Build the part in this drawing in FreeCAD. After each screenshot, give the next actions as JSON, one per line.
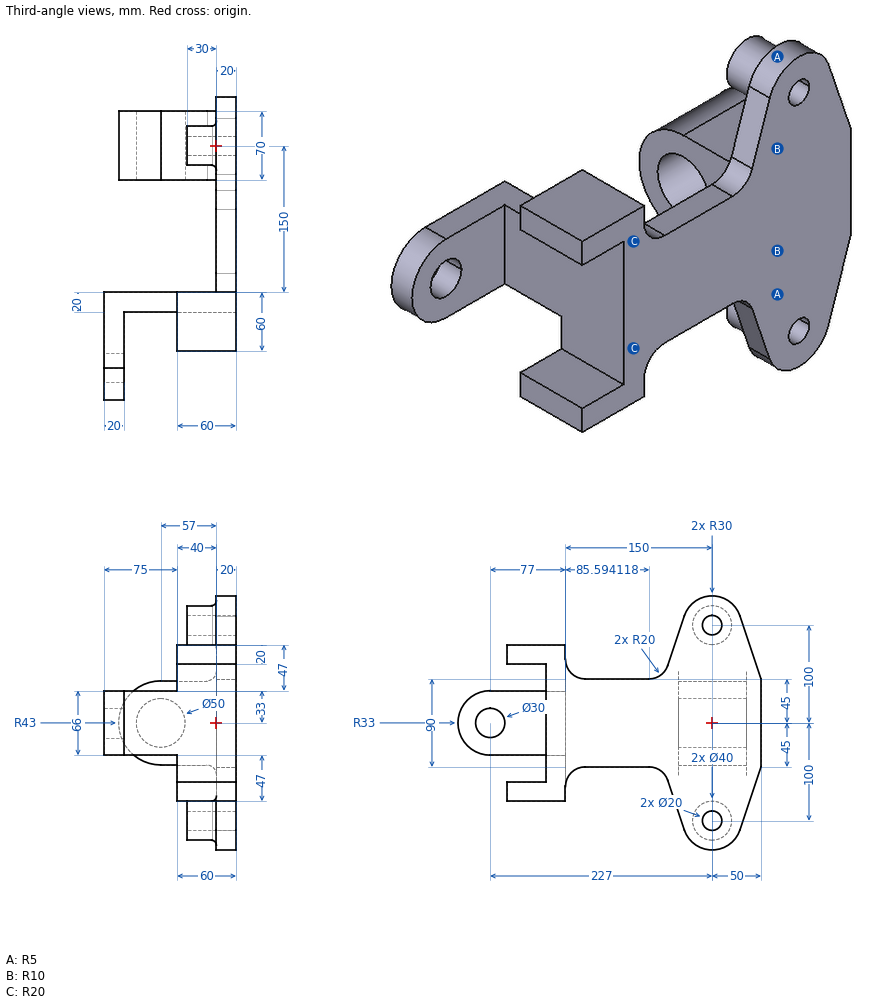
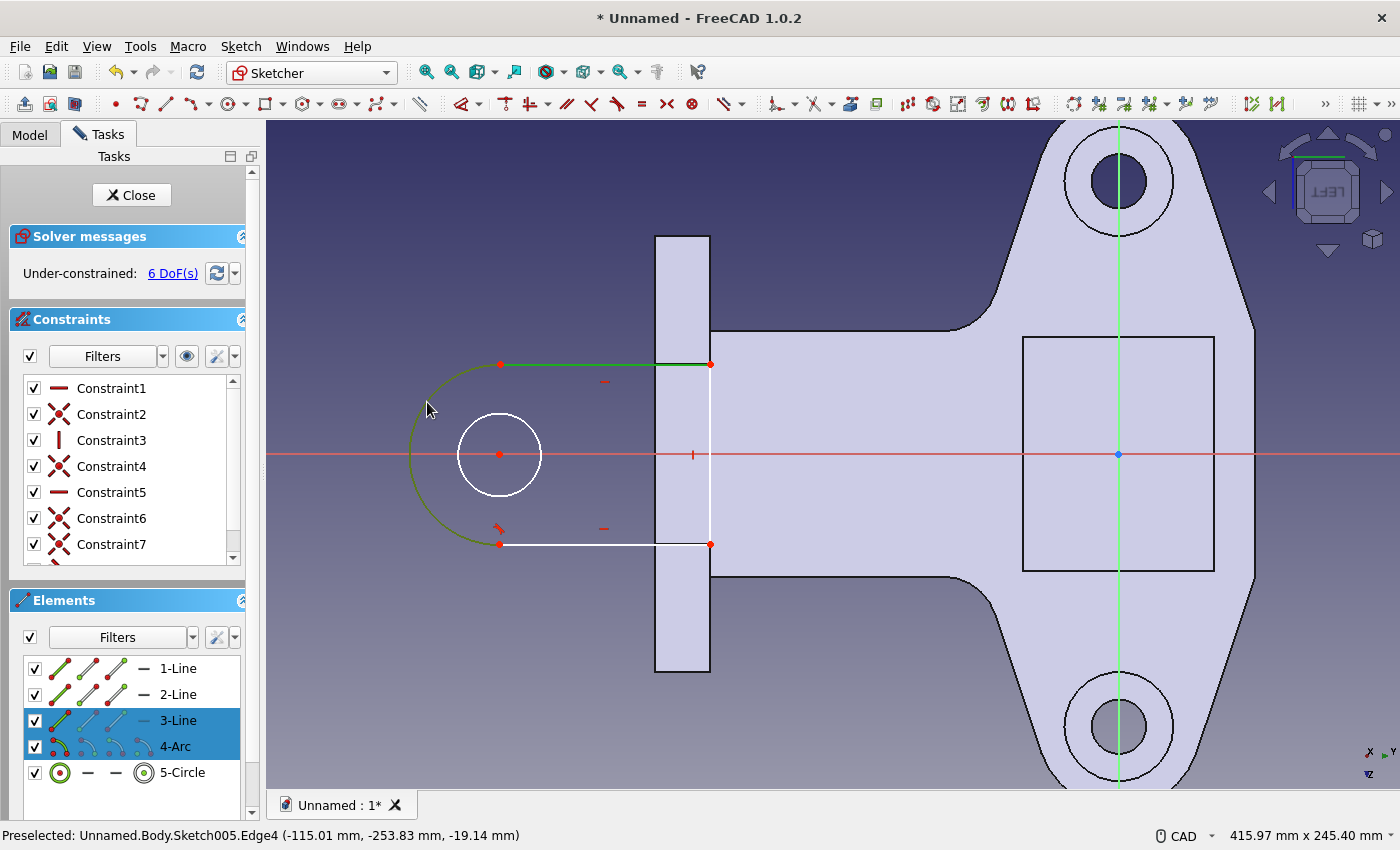
{"action": "left_click", "coordinate": [617, 104]}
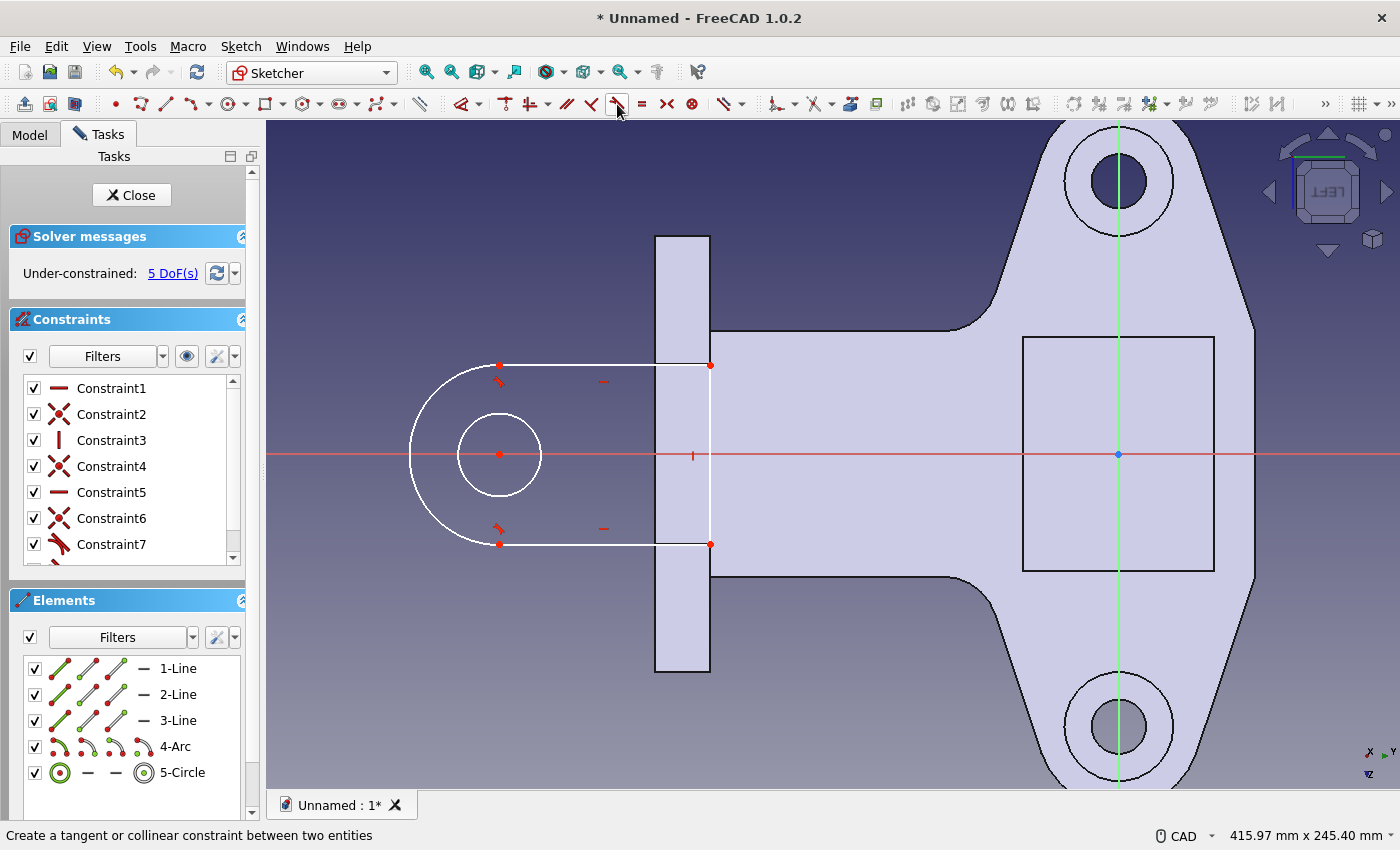
{"action": "left_click", "coordinate": [500, 455]}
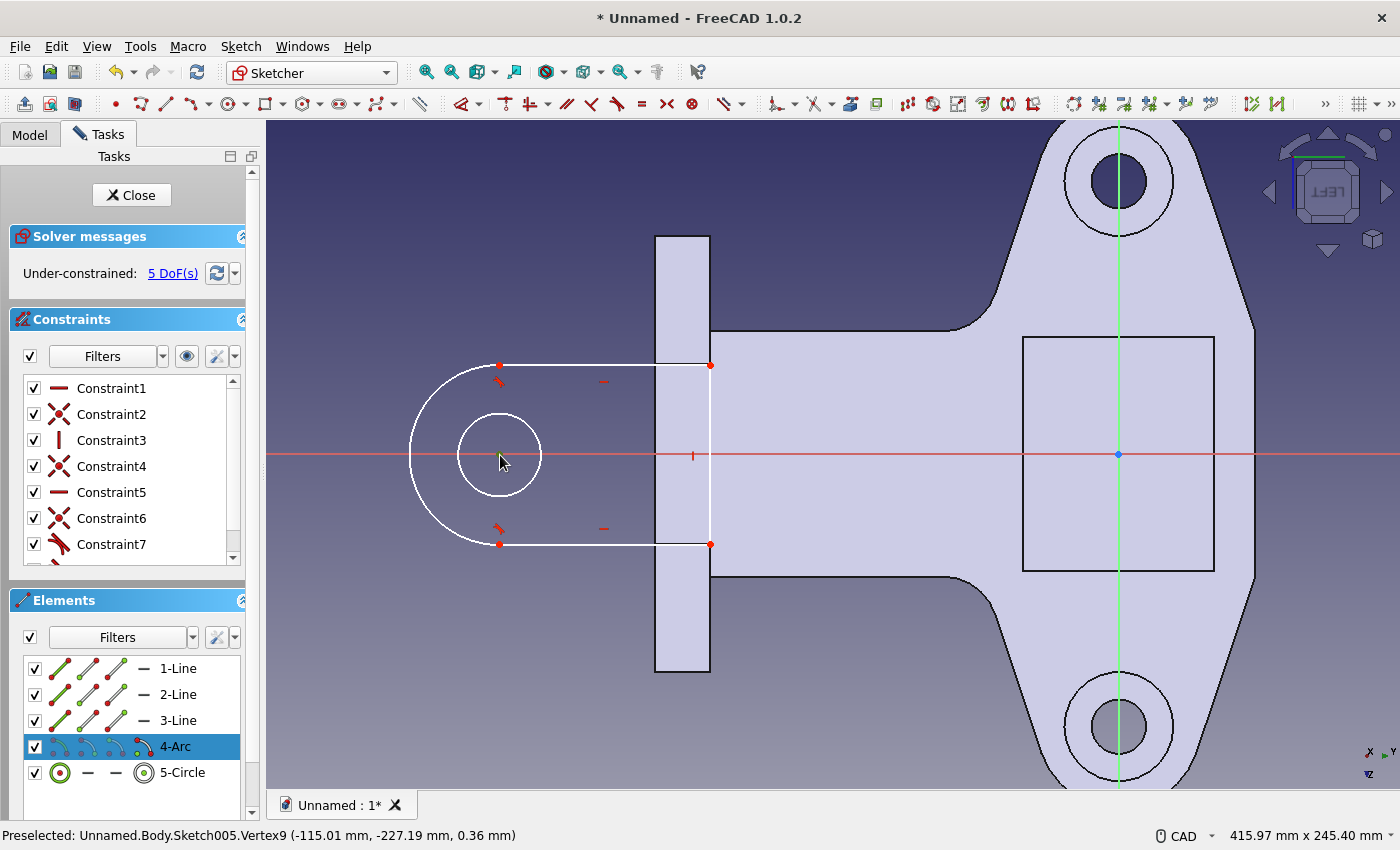
{"action": "left_click", "coordinate": [361, 454]}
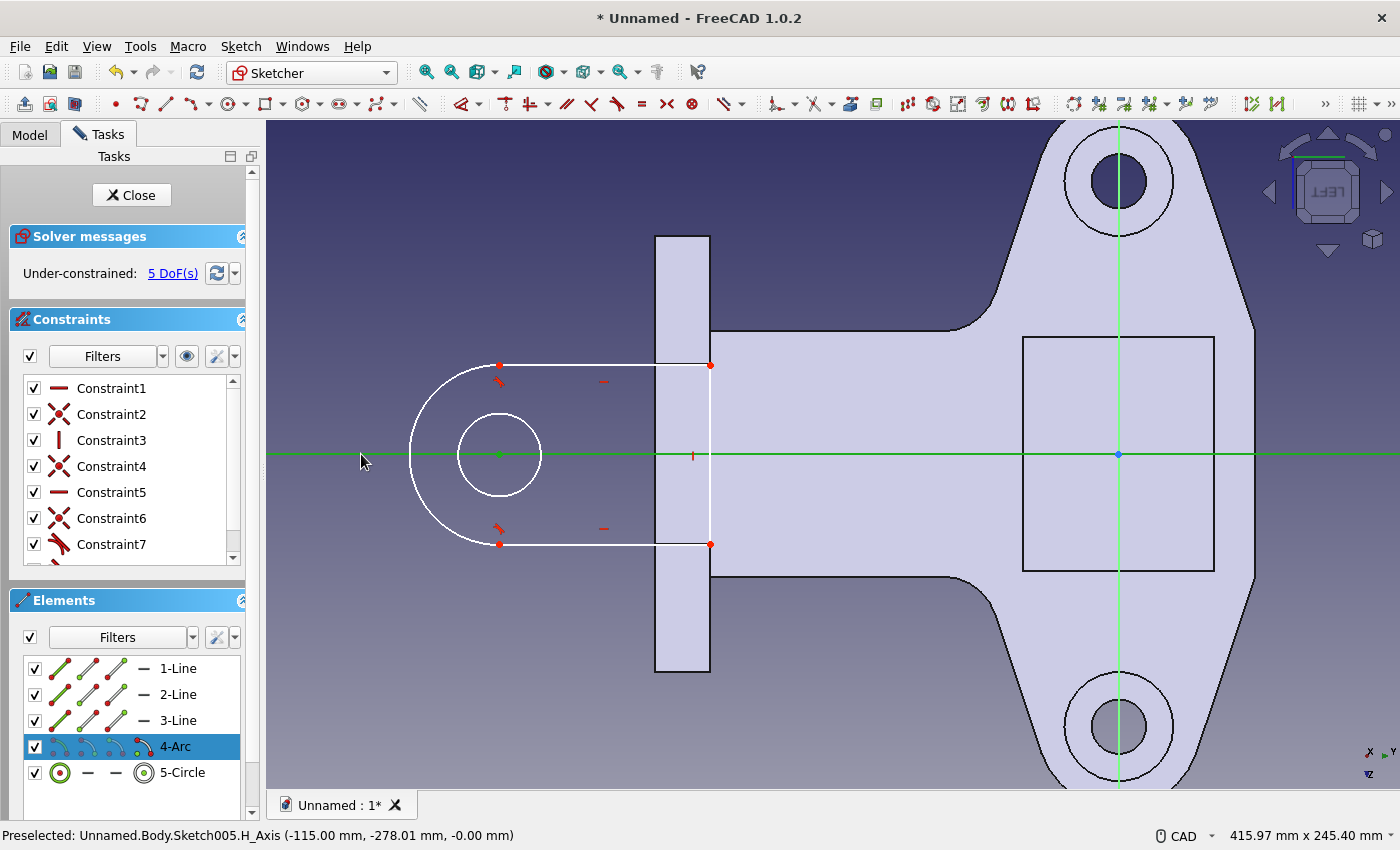
{"action": "left_click", "coordinate": [505, 104]}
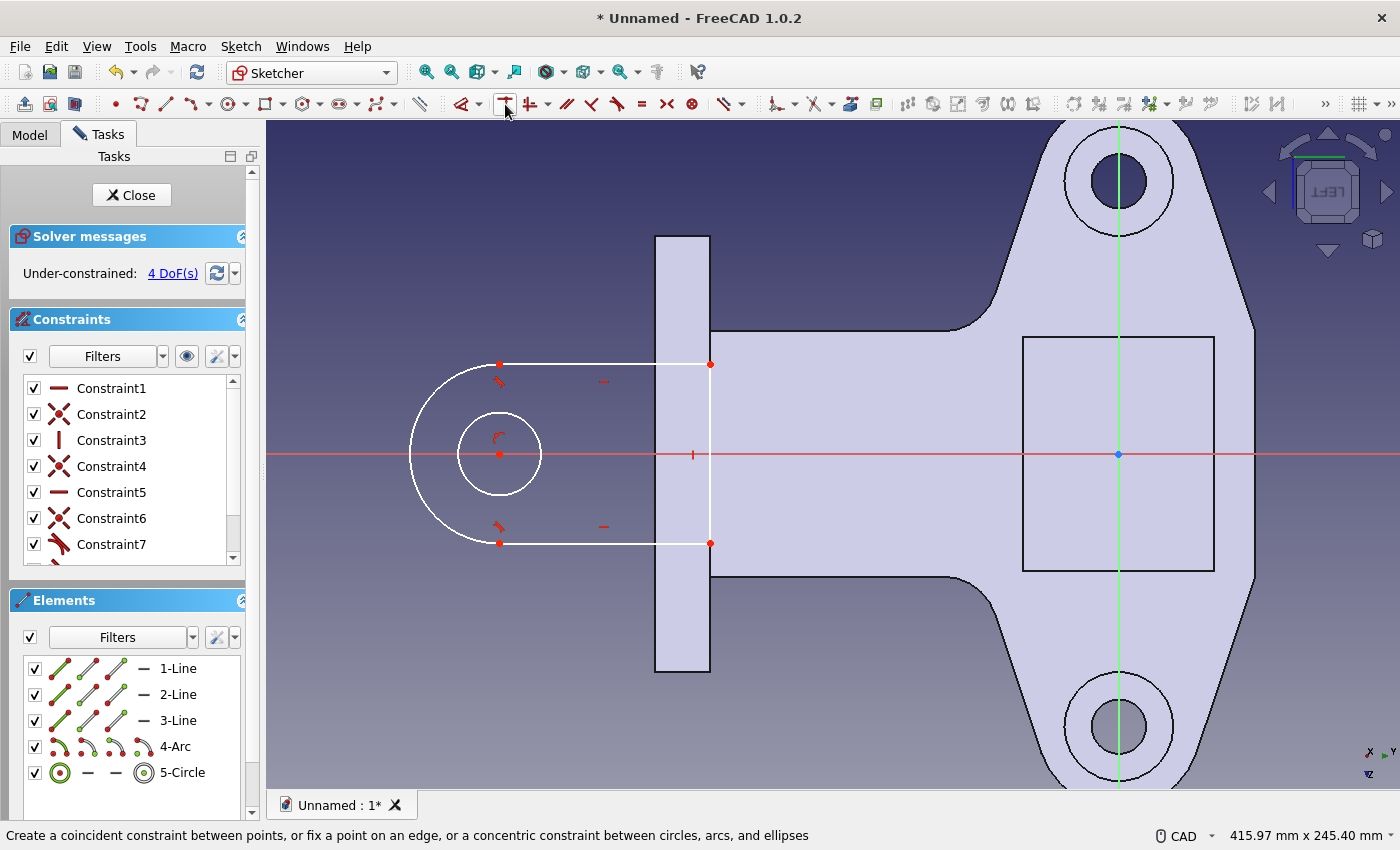
{"action": "key", "text": "d"}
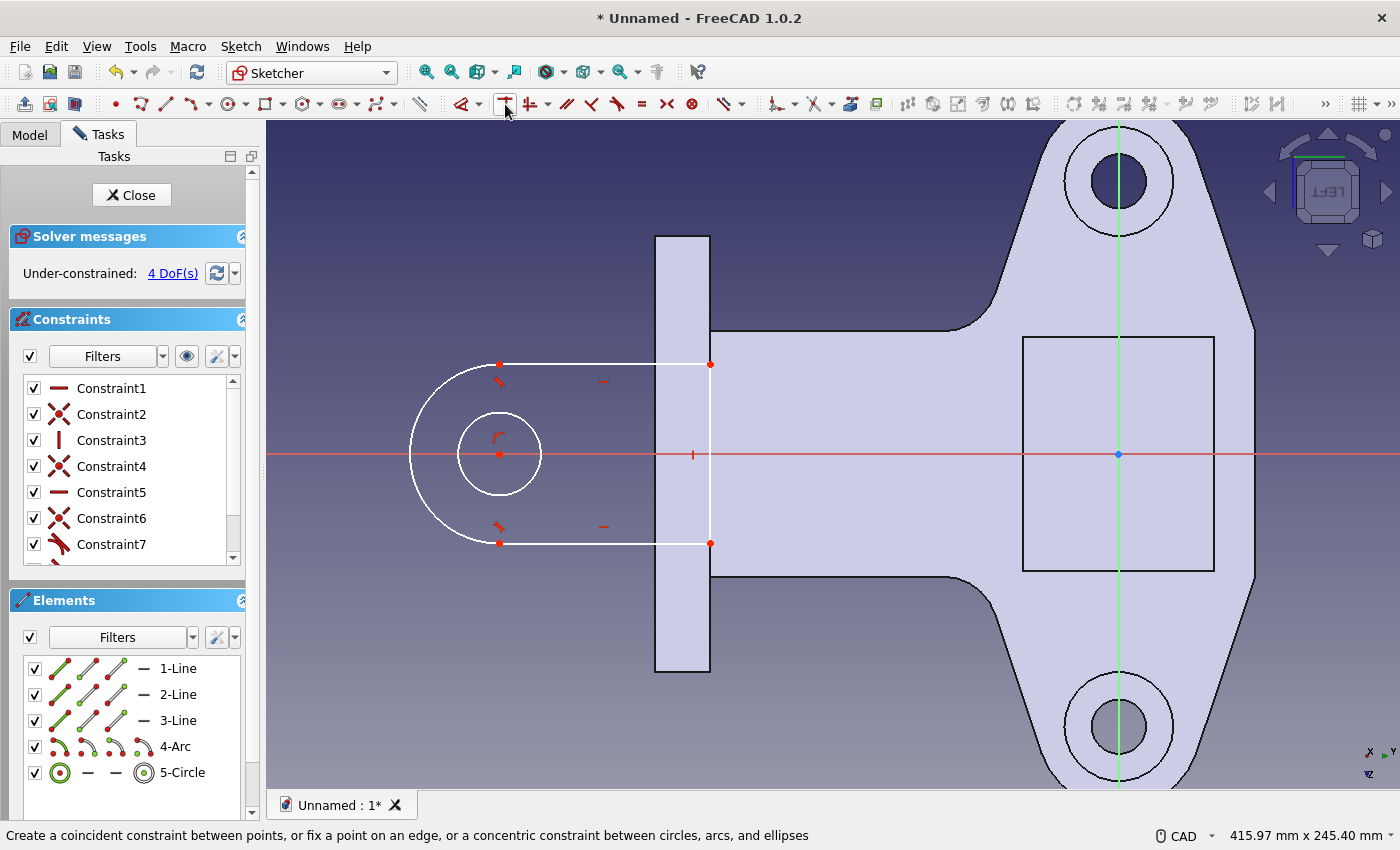
{"action": "left_click", "coordinate": [427, 401]}
{"action": "left_click", "coordinate": [401, 382]}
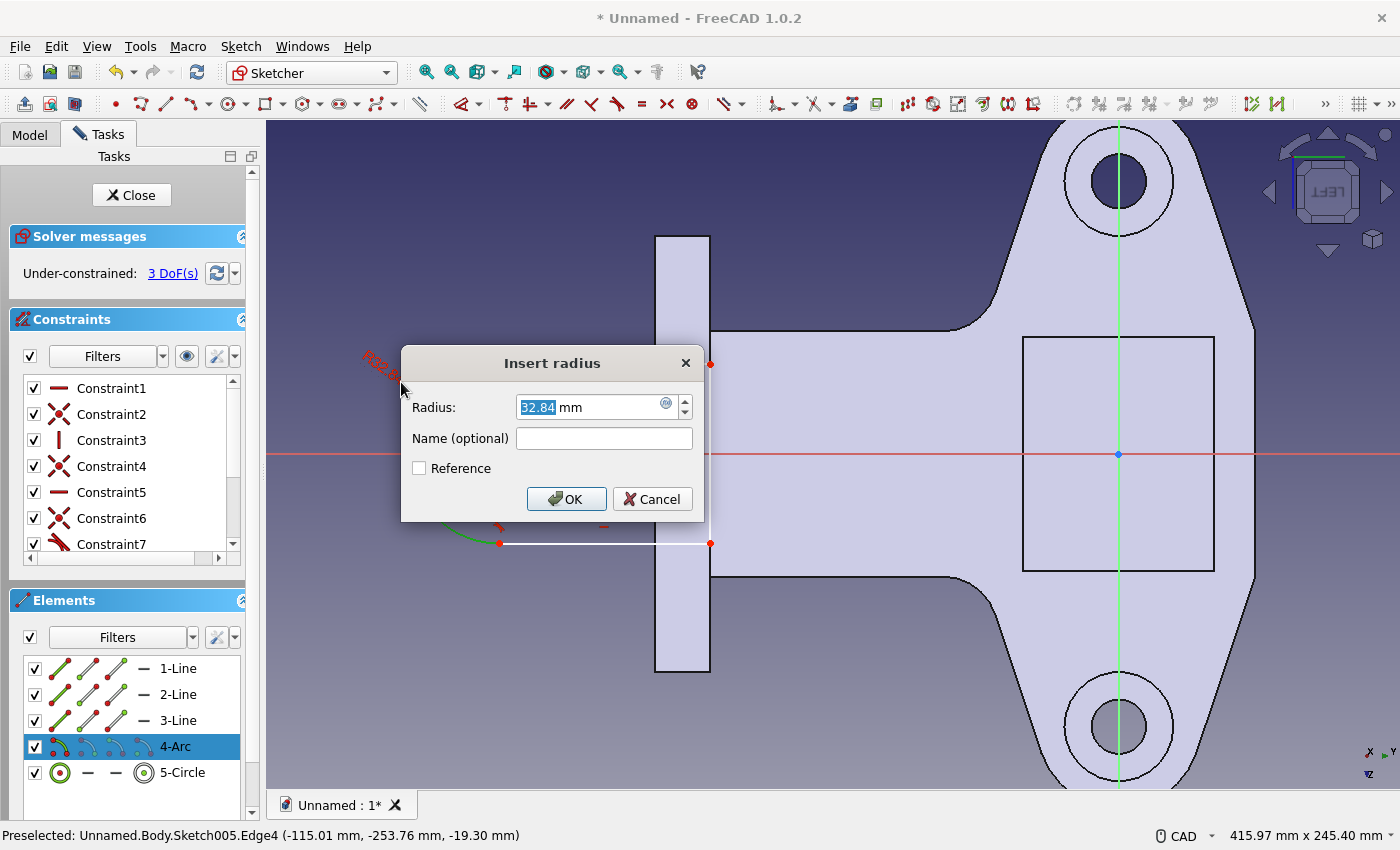
{"action": "type", "text": "33"}
{"action": "key", "text": "Return"}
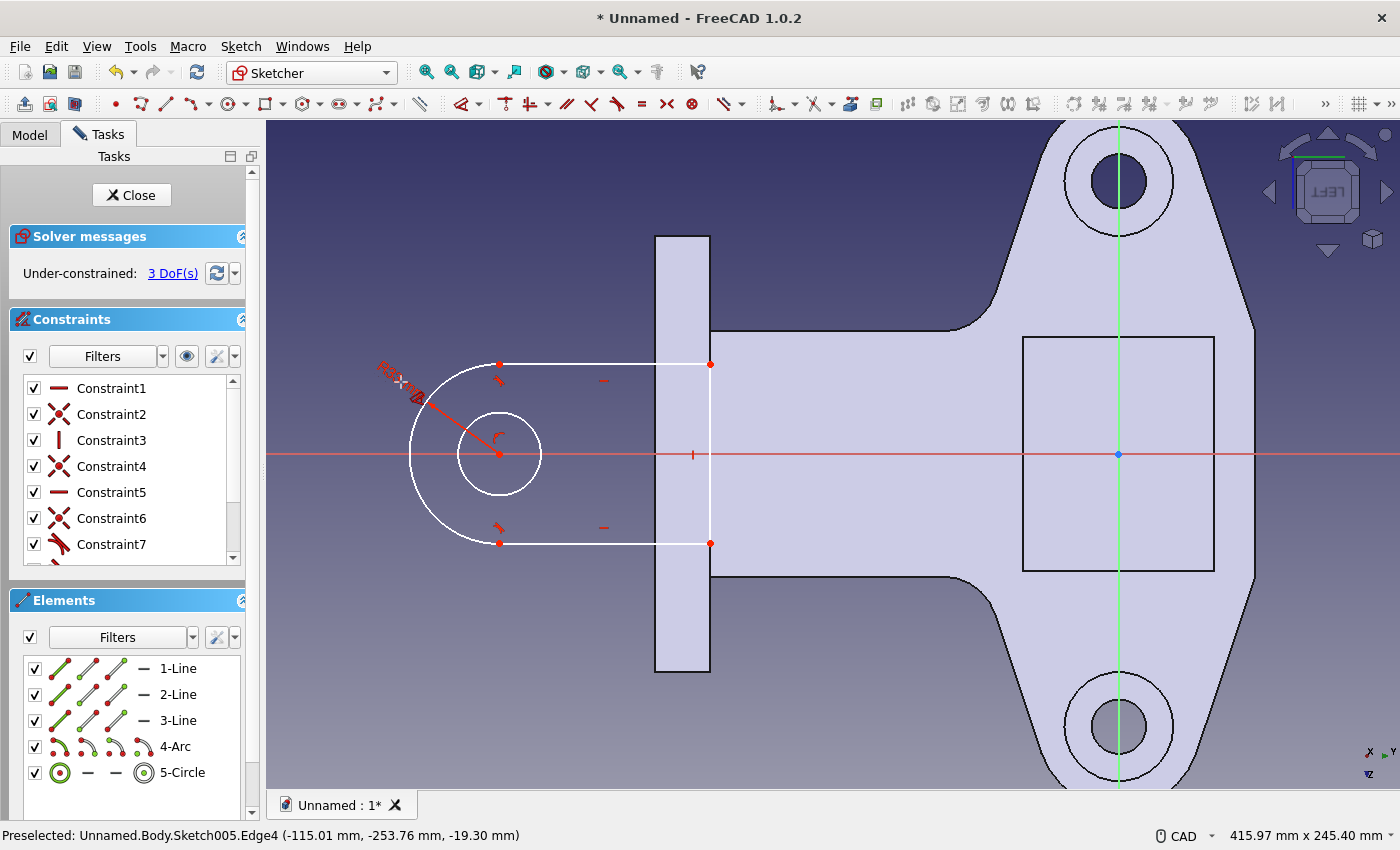
{"action": "left_click", "coordinate": [529, 425]}
{"action": "left_click", "coordinate": [552, 403]}